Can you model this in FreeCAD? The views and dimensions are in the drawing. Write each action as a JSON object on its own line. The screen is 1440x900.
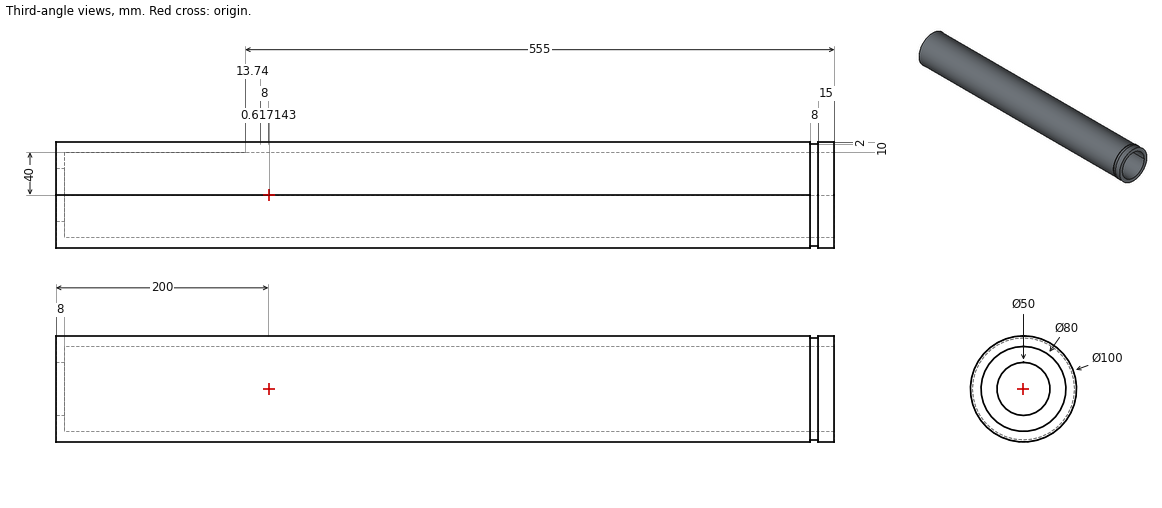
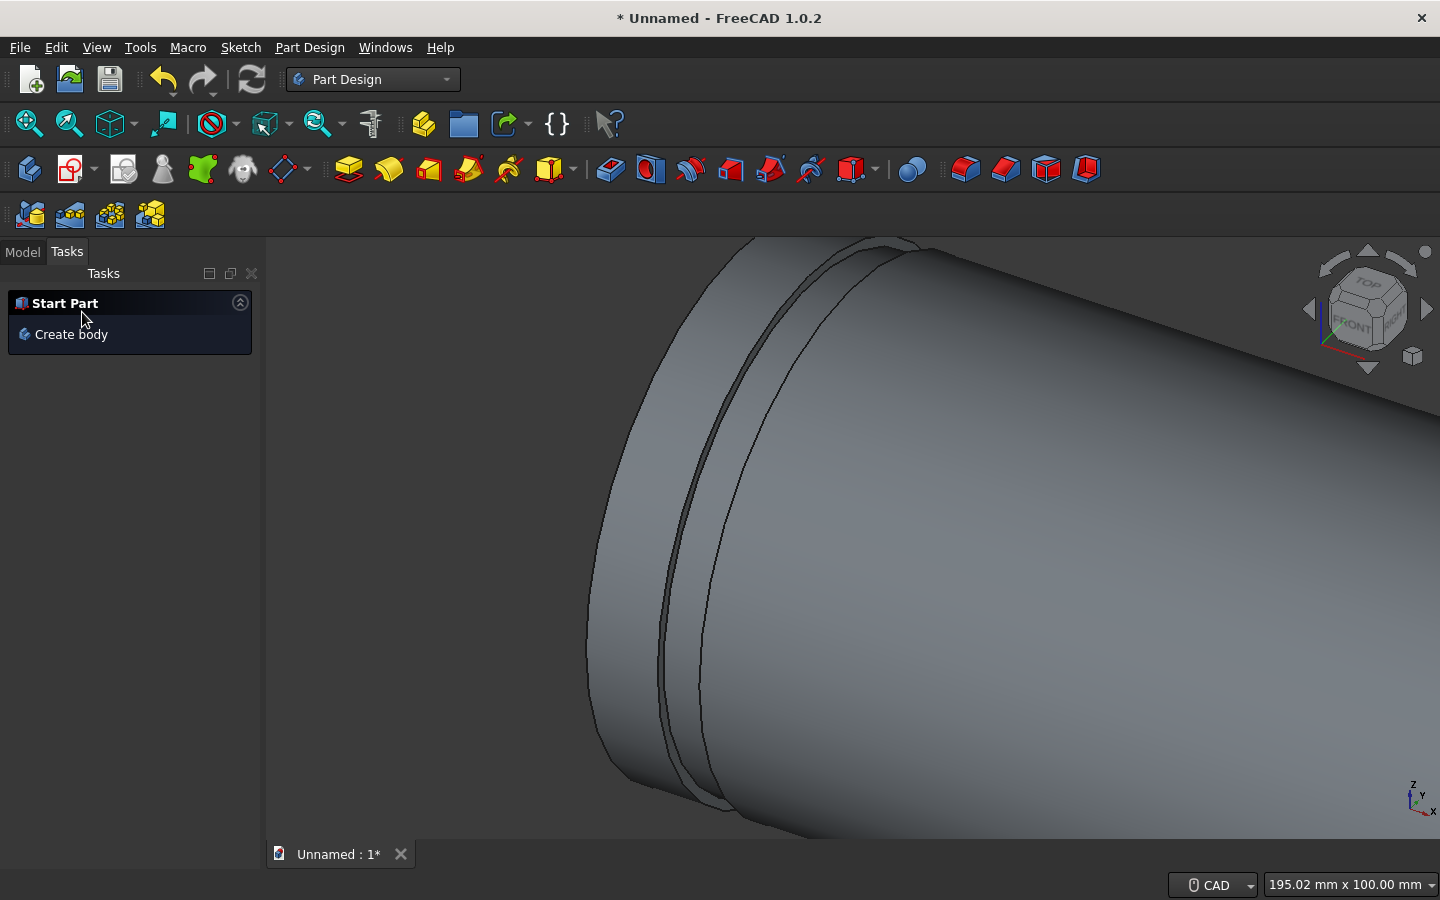
{"action": "key", "text": "v f"}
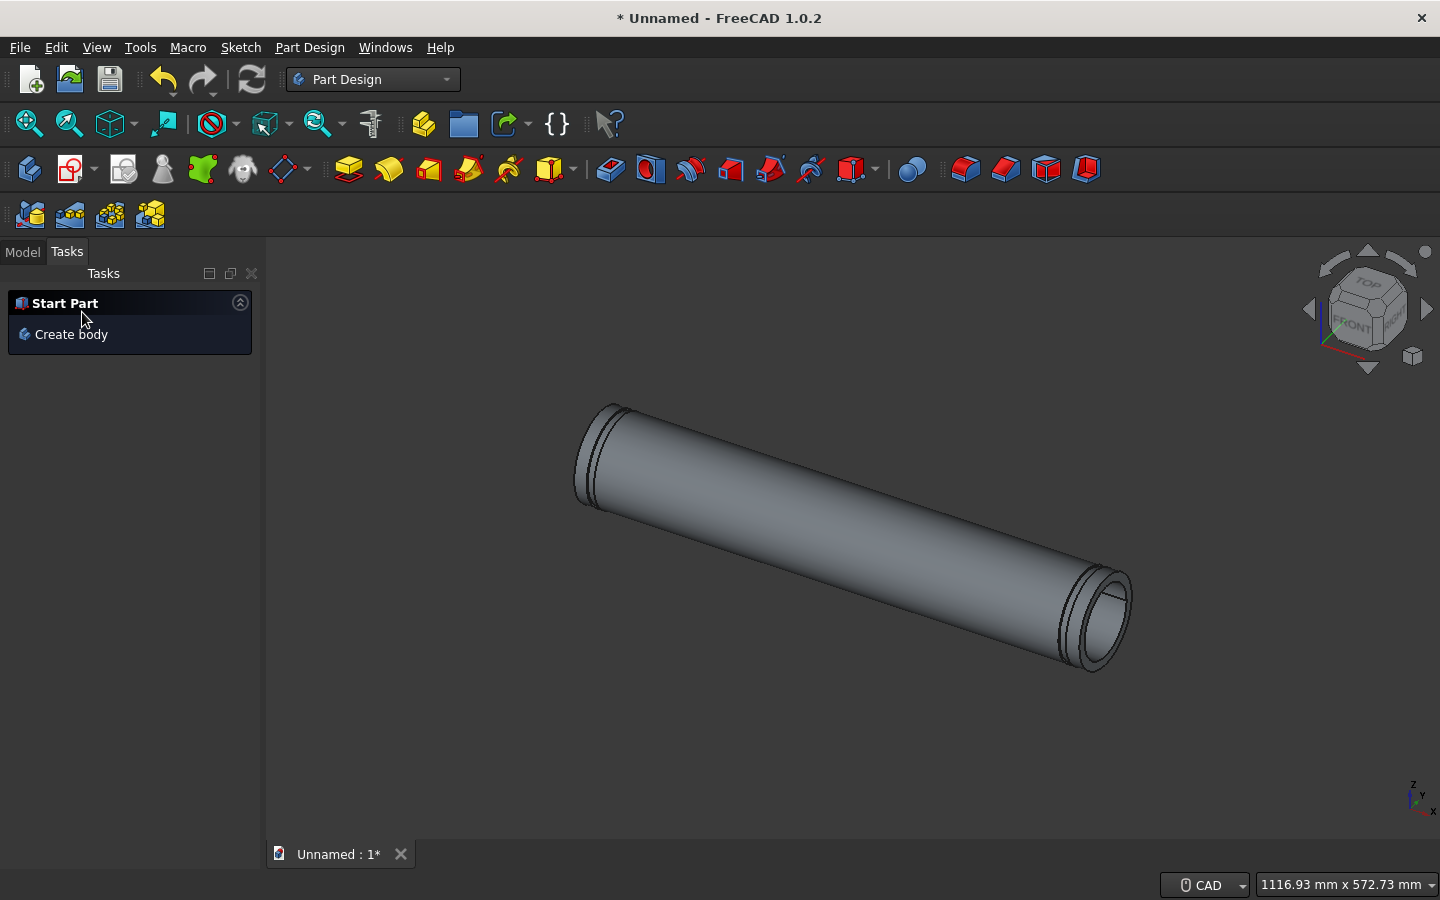
{"action": "left_click", "coordinate": [23, 251]}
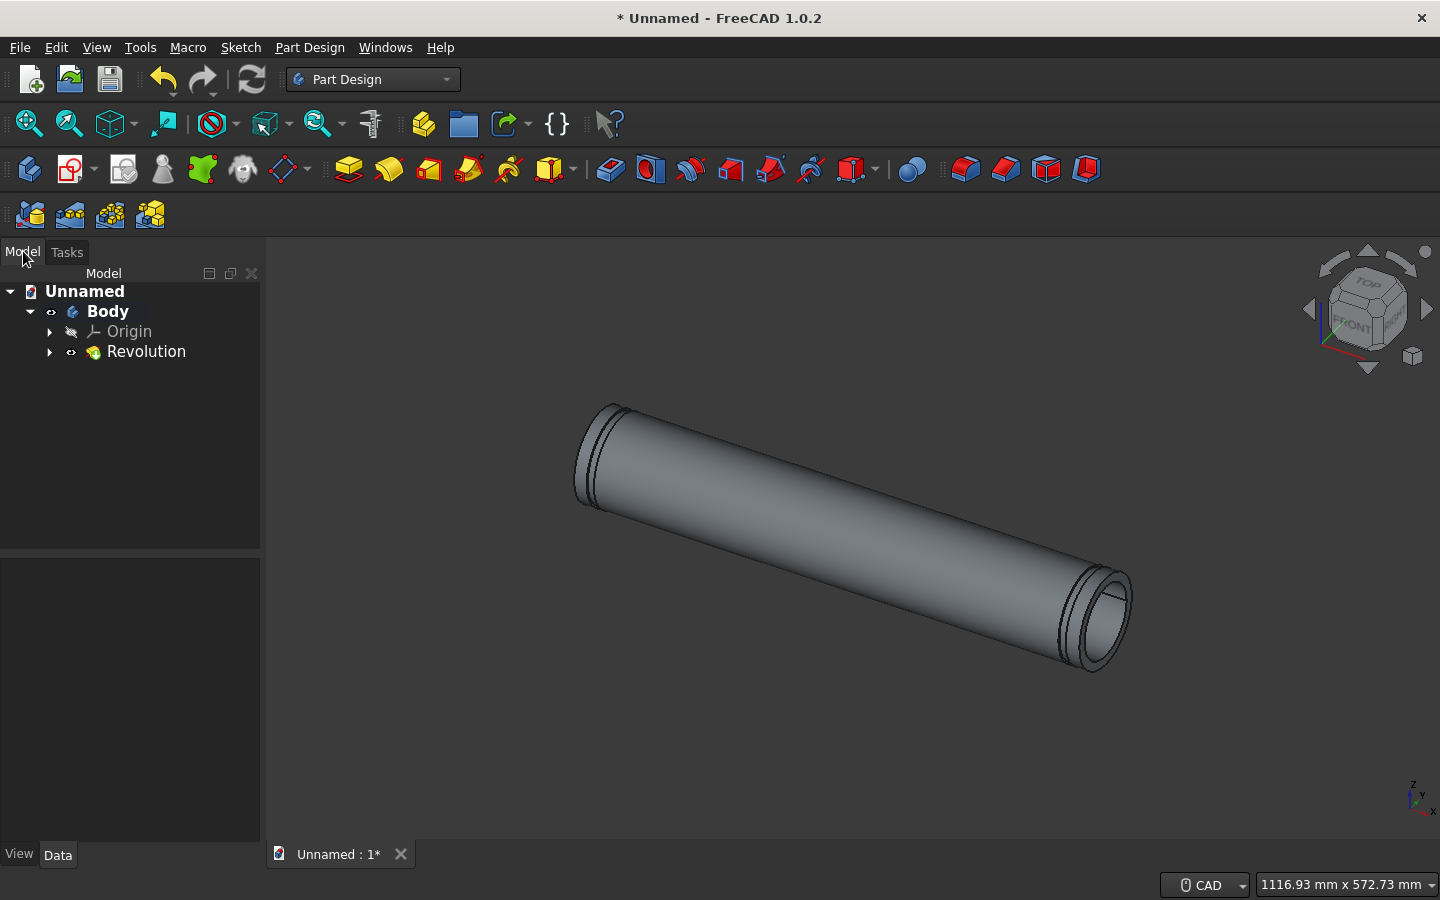
{"action": "left_click", "coordinate": [50, 332]}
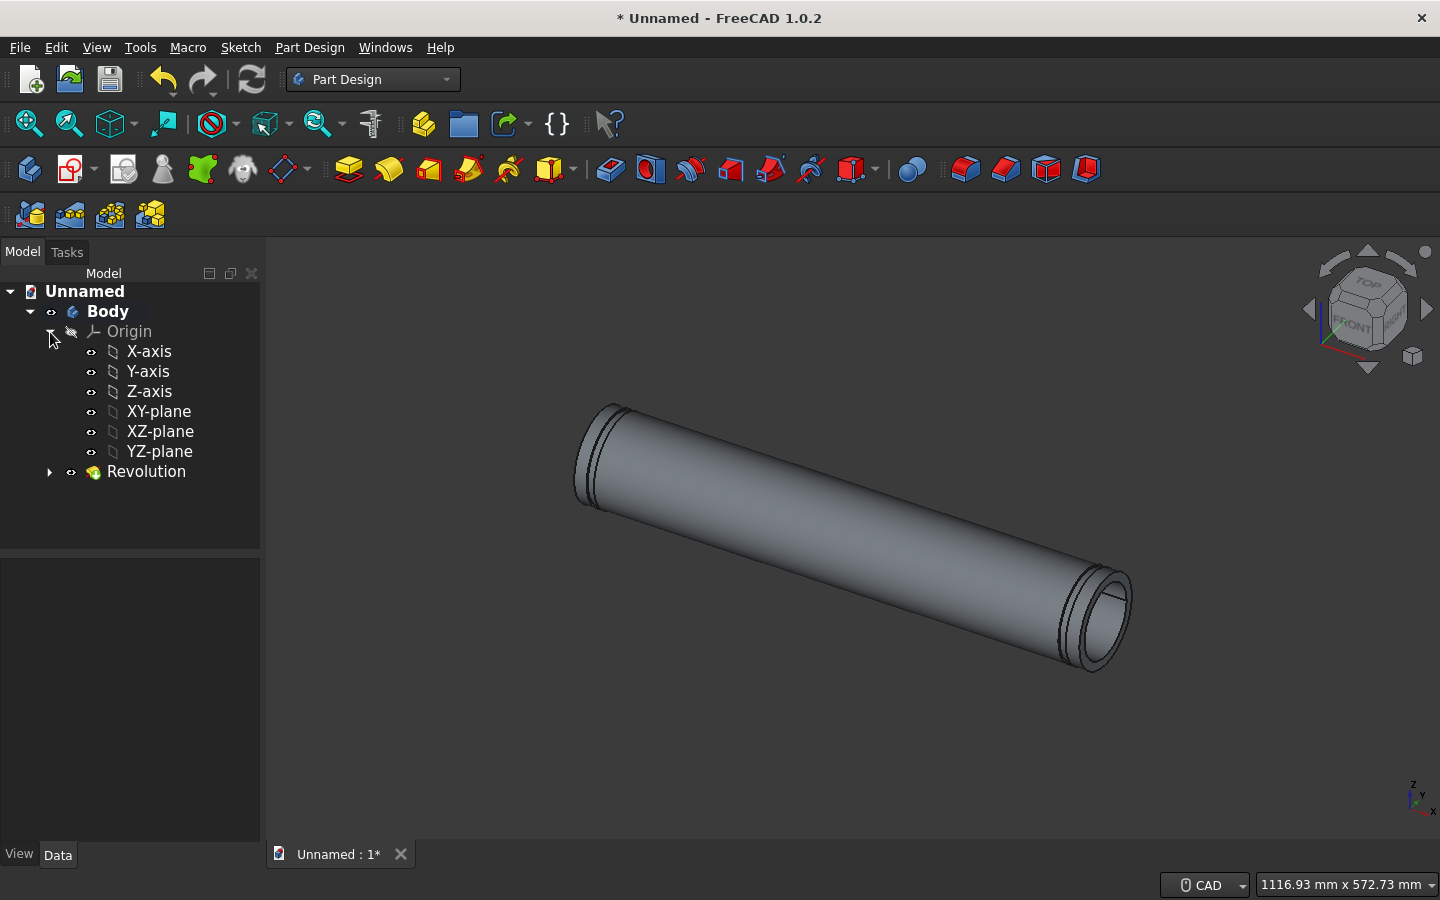
{"action": "left_click", "coordinate": [136, 452]}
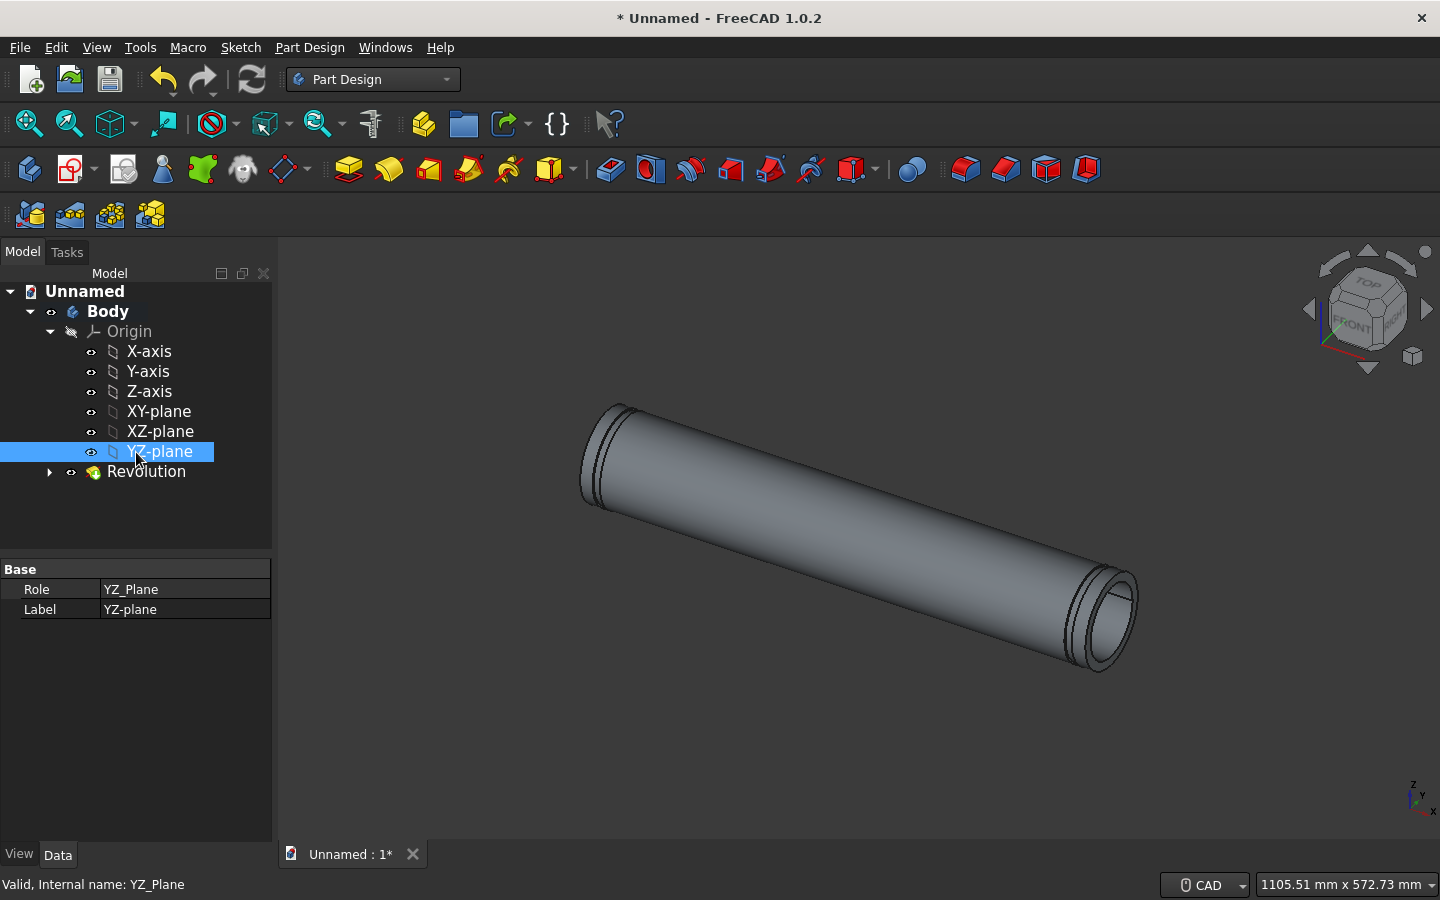
{"action": "left_click", "coordinate": [284, 170]}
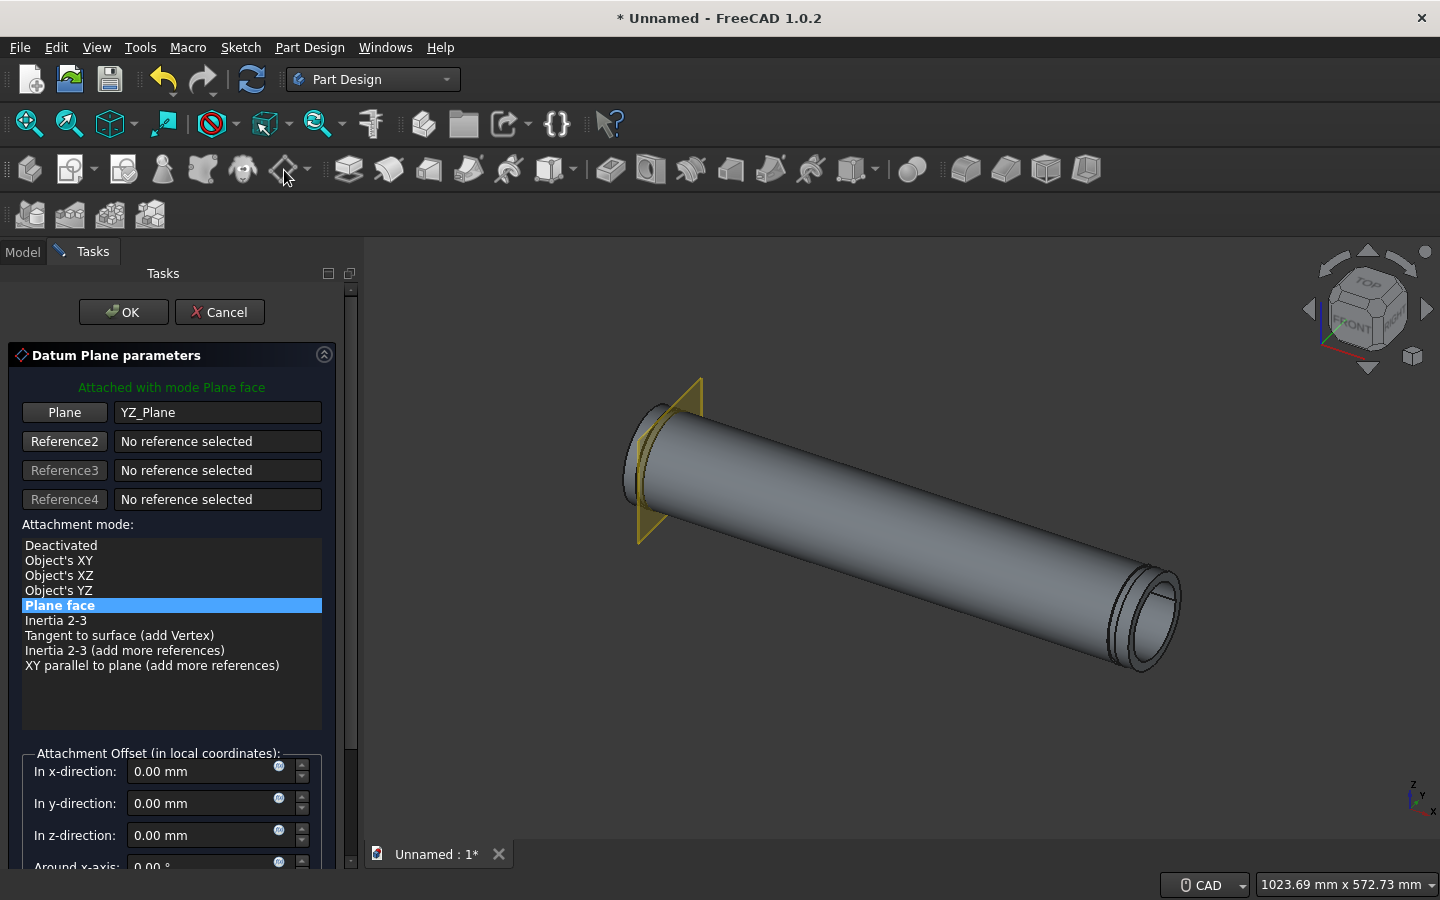
{"action": "triple_click", "coordinate": [210, 835]}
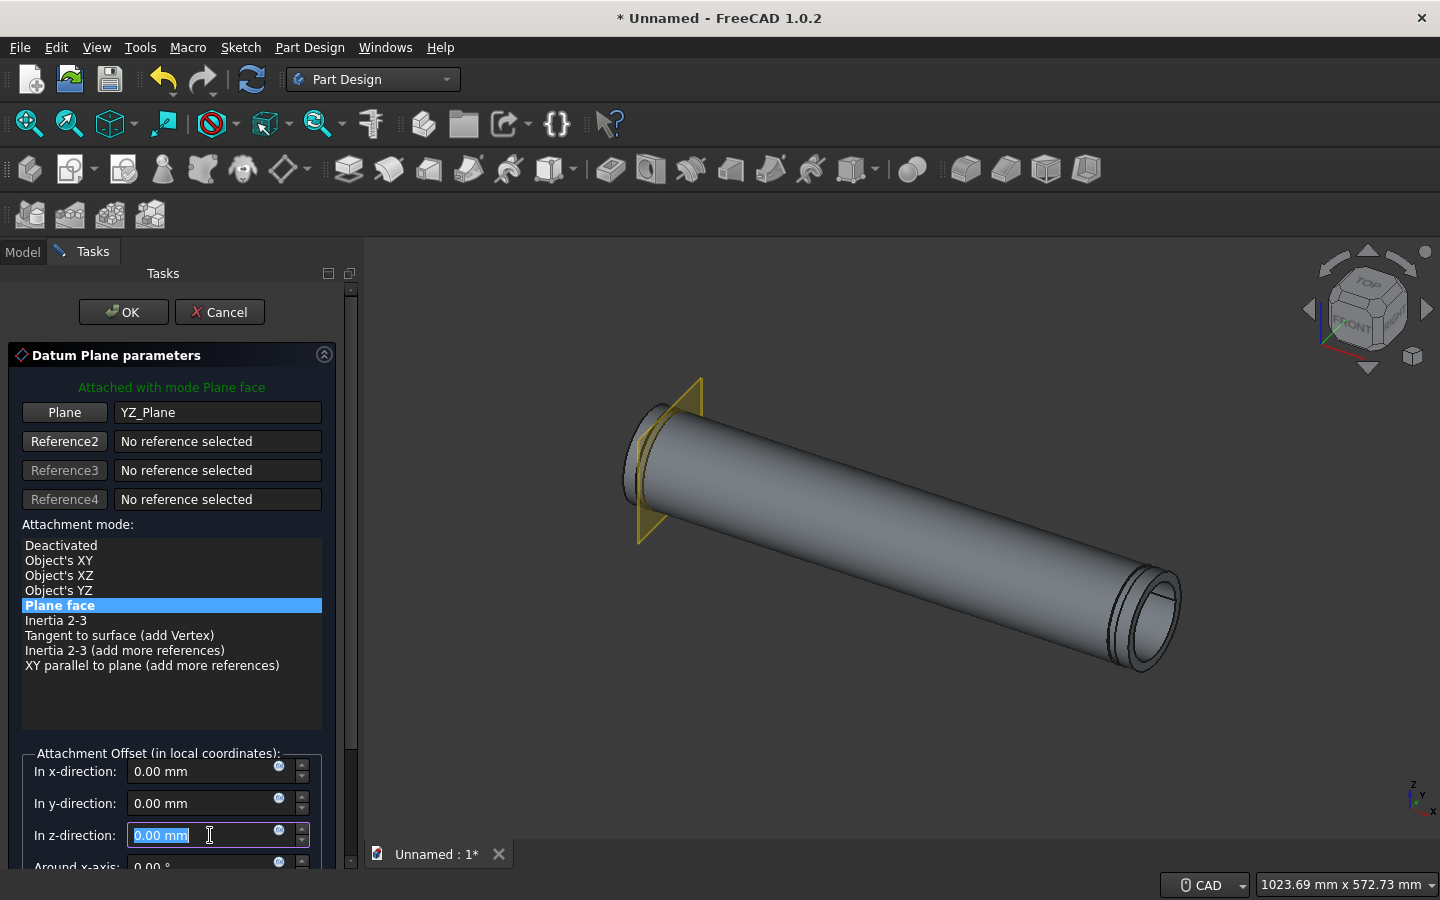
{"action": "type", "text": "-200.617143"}
{"action": "key", "text": "Tab"}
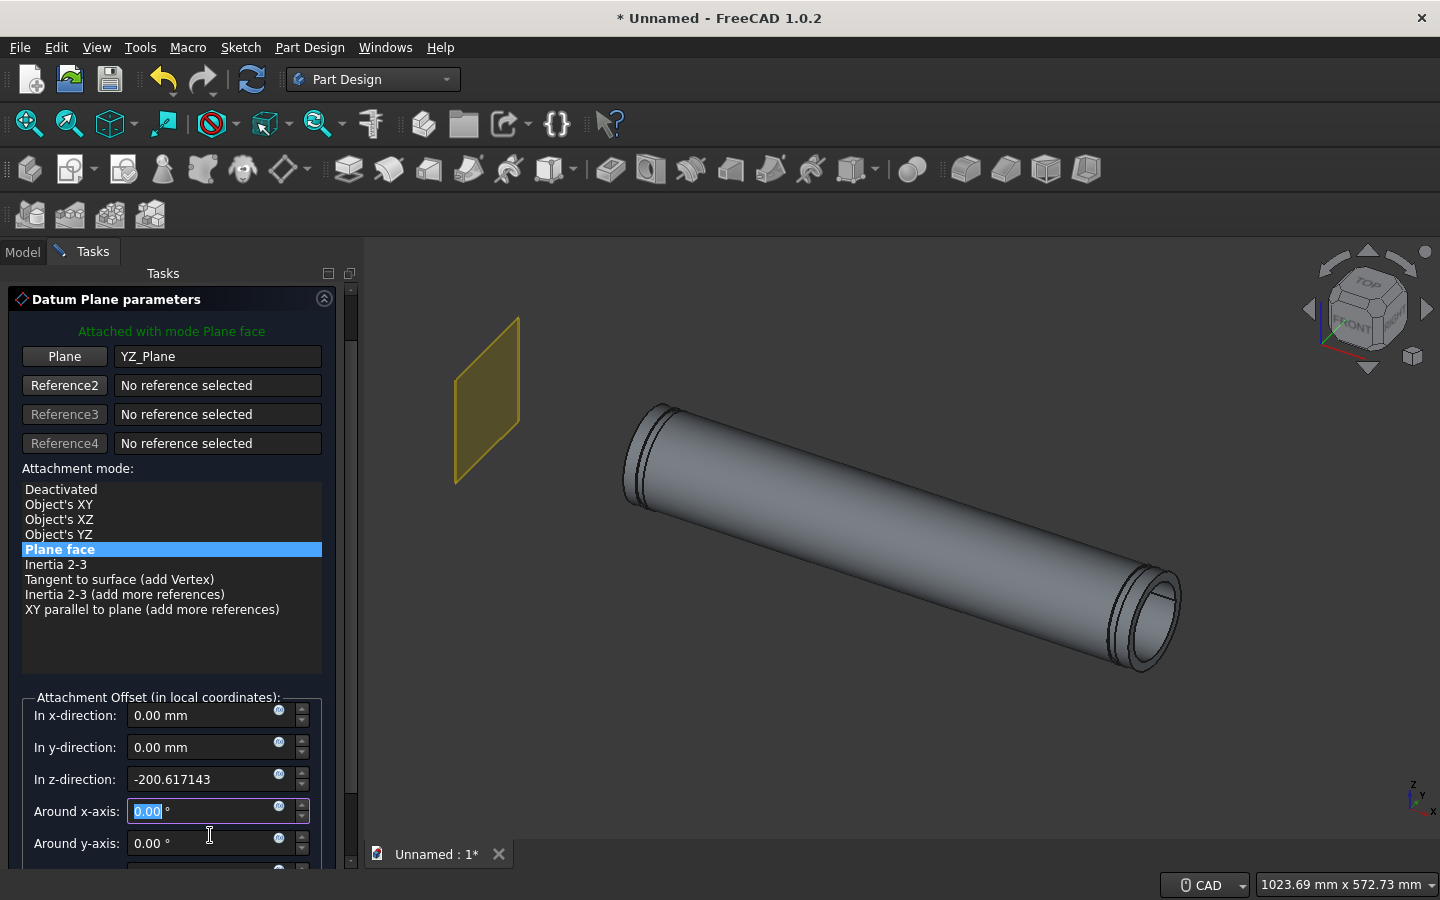
{"action": "scroll", "coordinate": [351, 576], "scroll_direction": "up", "scroll_amount": 2}